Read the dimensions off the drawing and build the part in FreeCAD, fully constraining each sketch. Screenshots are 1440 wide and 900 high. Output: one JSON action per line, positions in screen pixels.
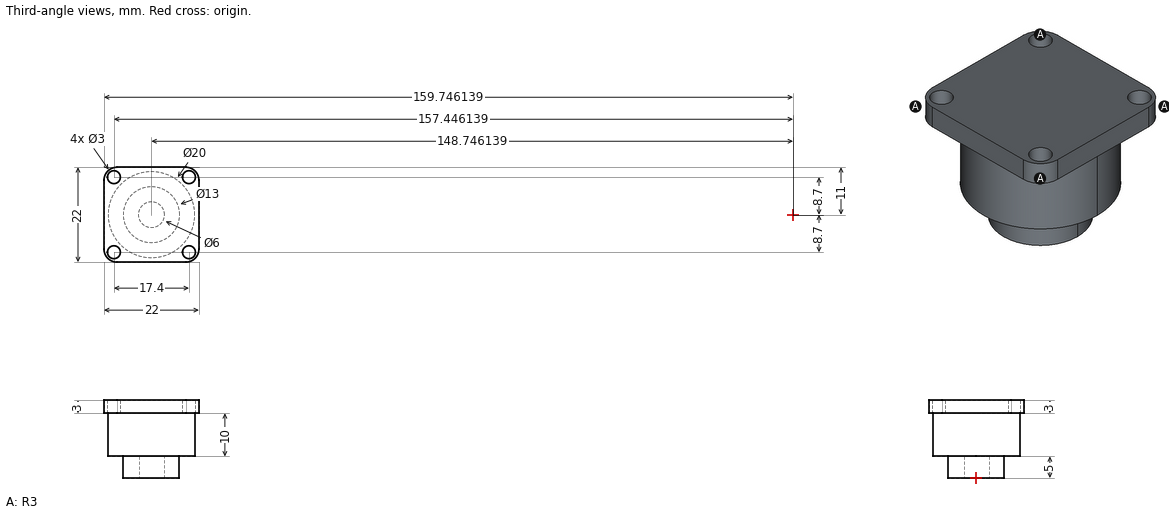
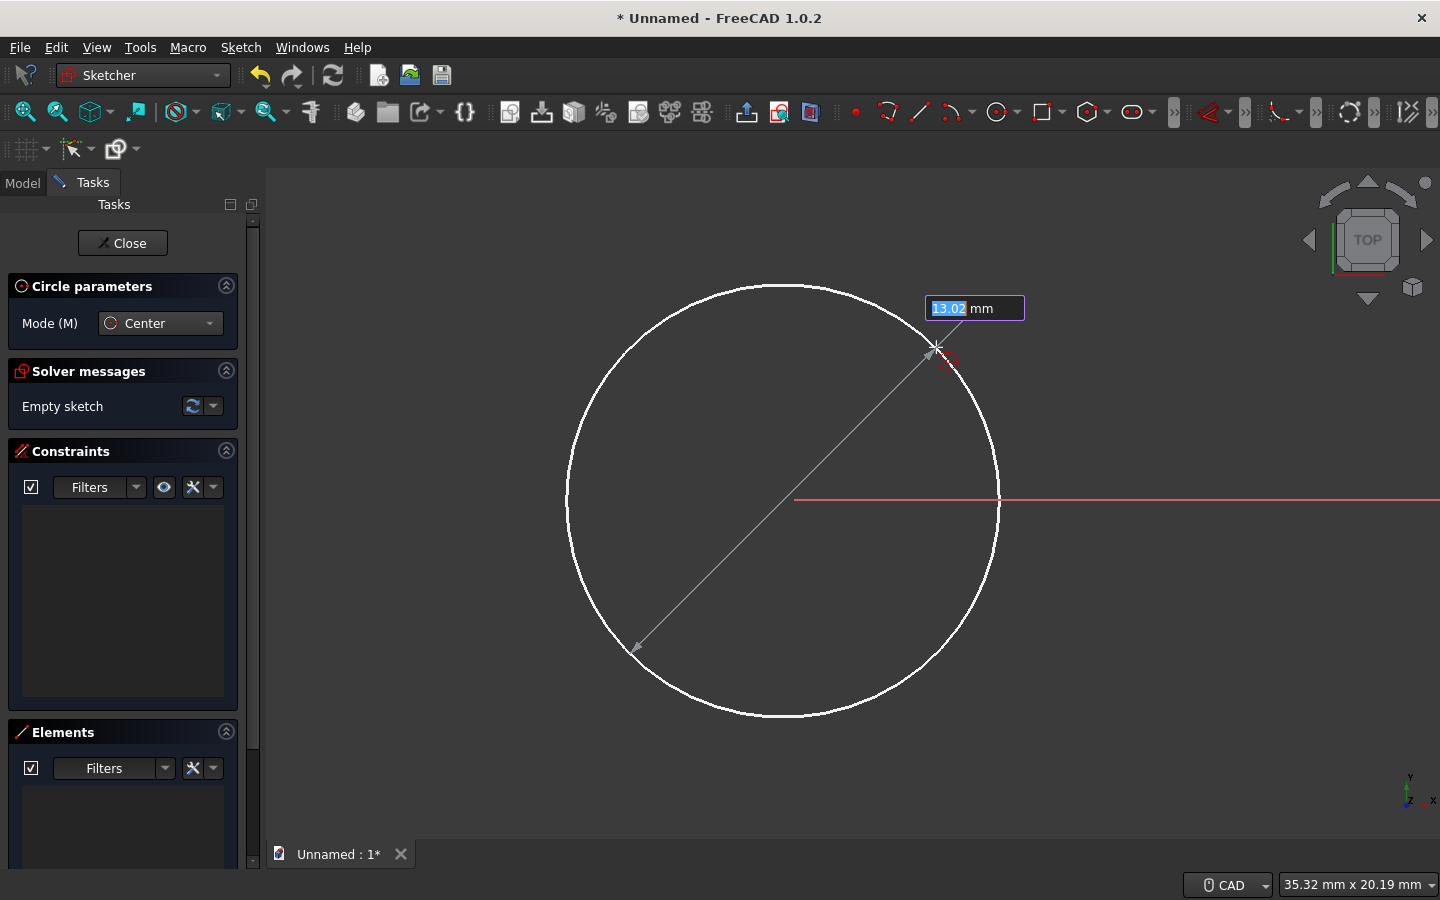
{"action": "type", "text": "13"}
{"action": "key", "text": "Return"}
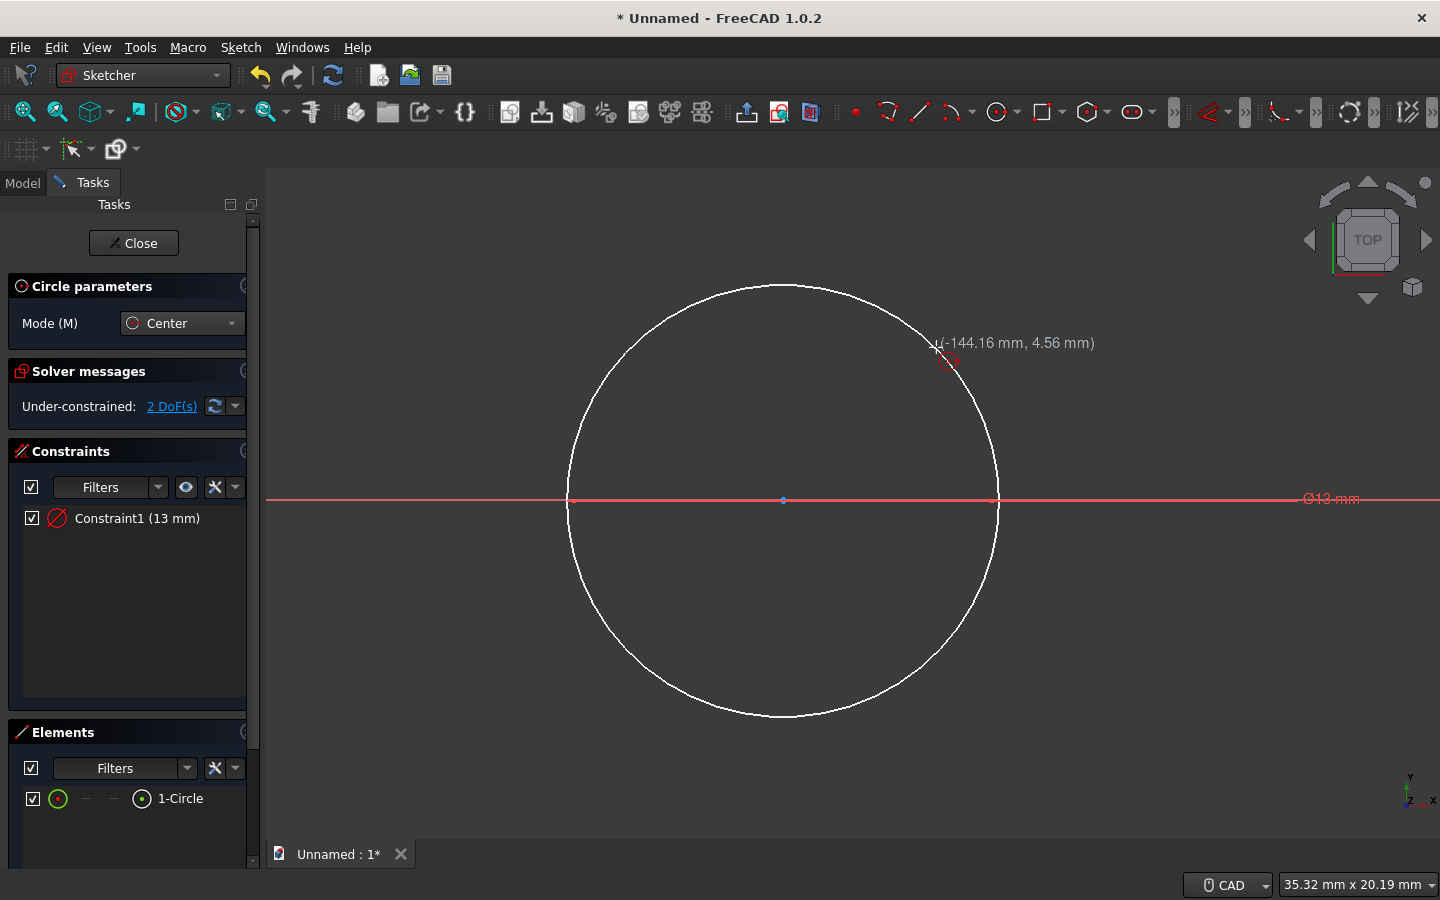
{"action": "left_click", "coordinate": [783, 501]}
{"action": "mouse_move", "coordinate": [854, 429]}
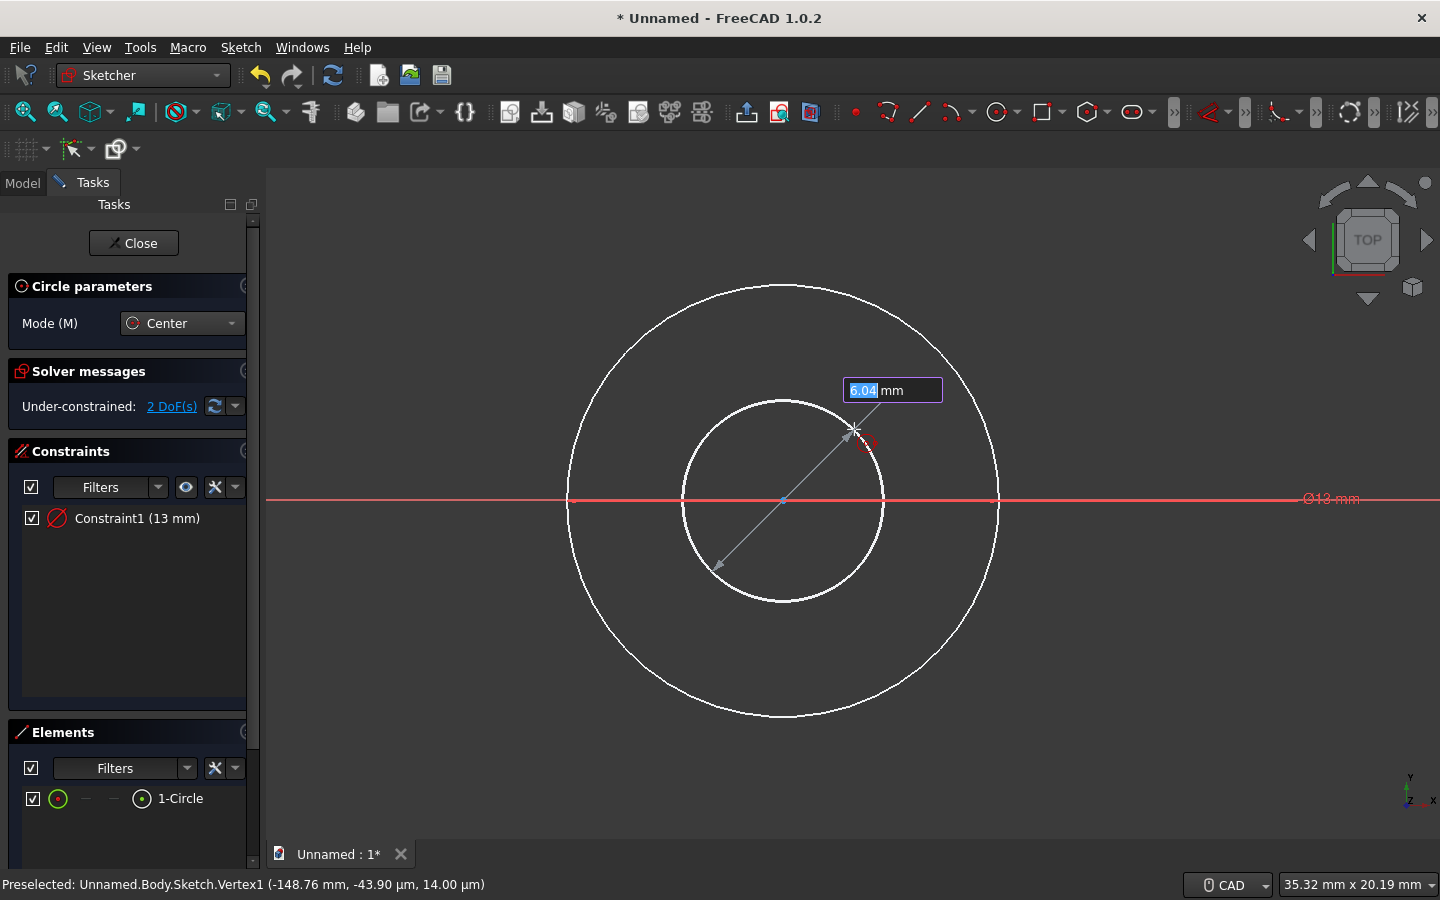
{"action": "type", "text": "6"}
{"action": "key", "text": "Return"}
{"action": "key", "text": "Escape"}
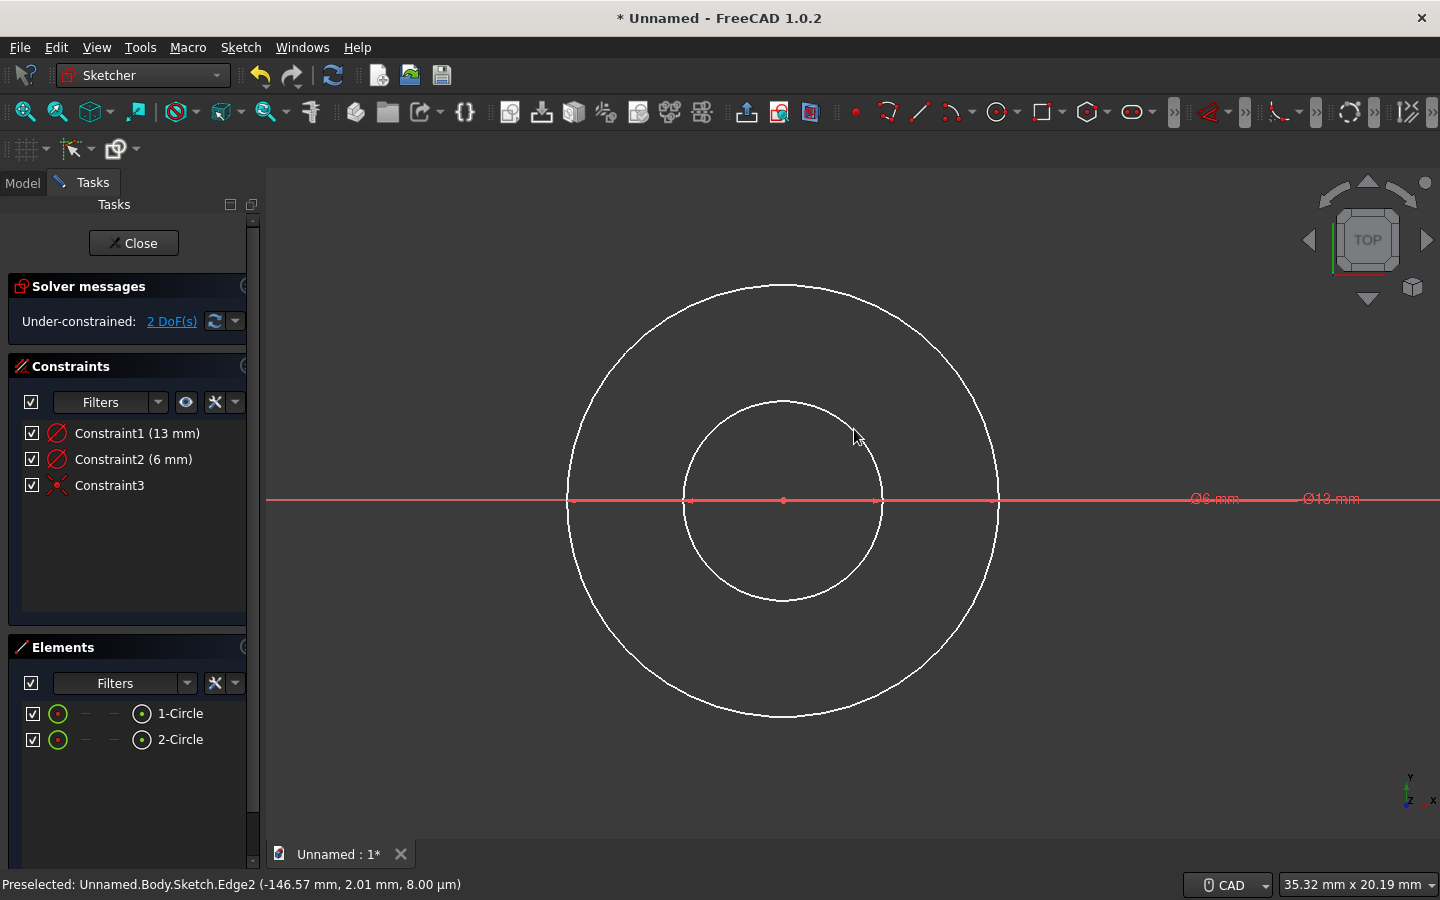
{"action": "left_click", "coordinate": [783, 501]}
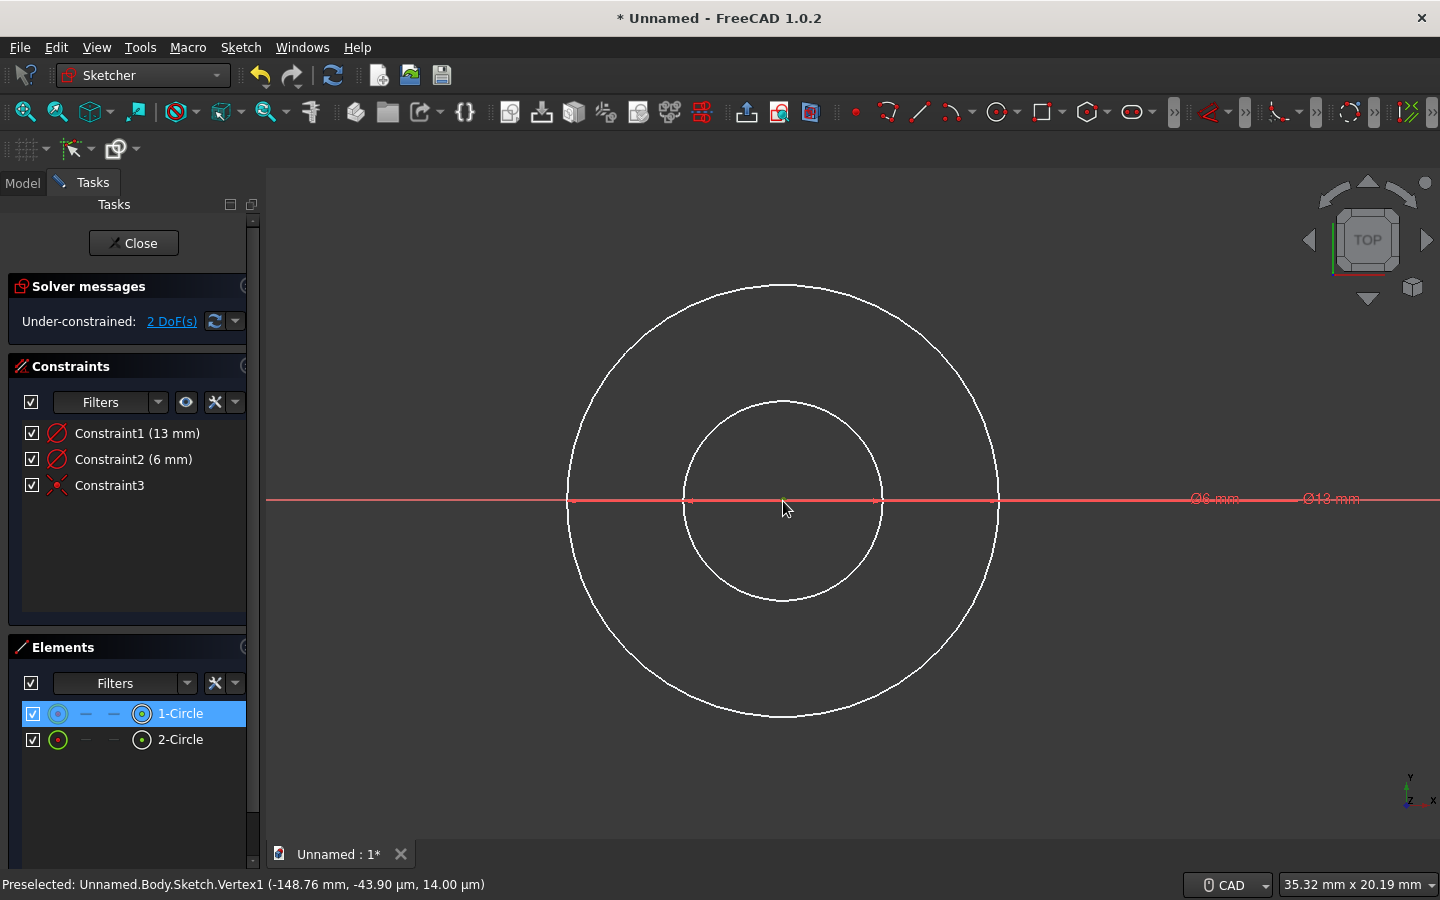
{"action": "left_click", "coordinate": [364, 500]}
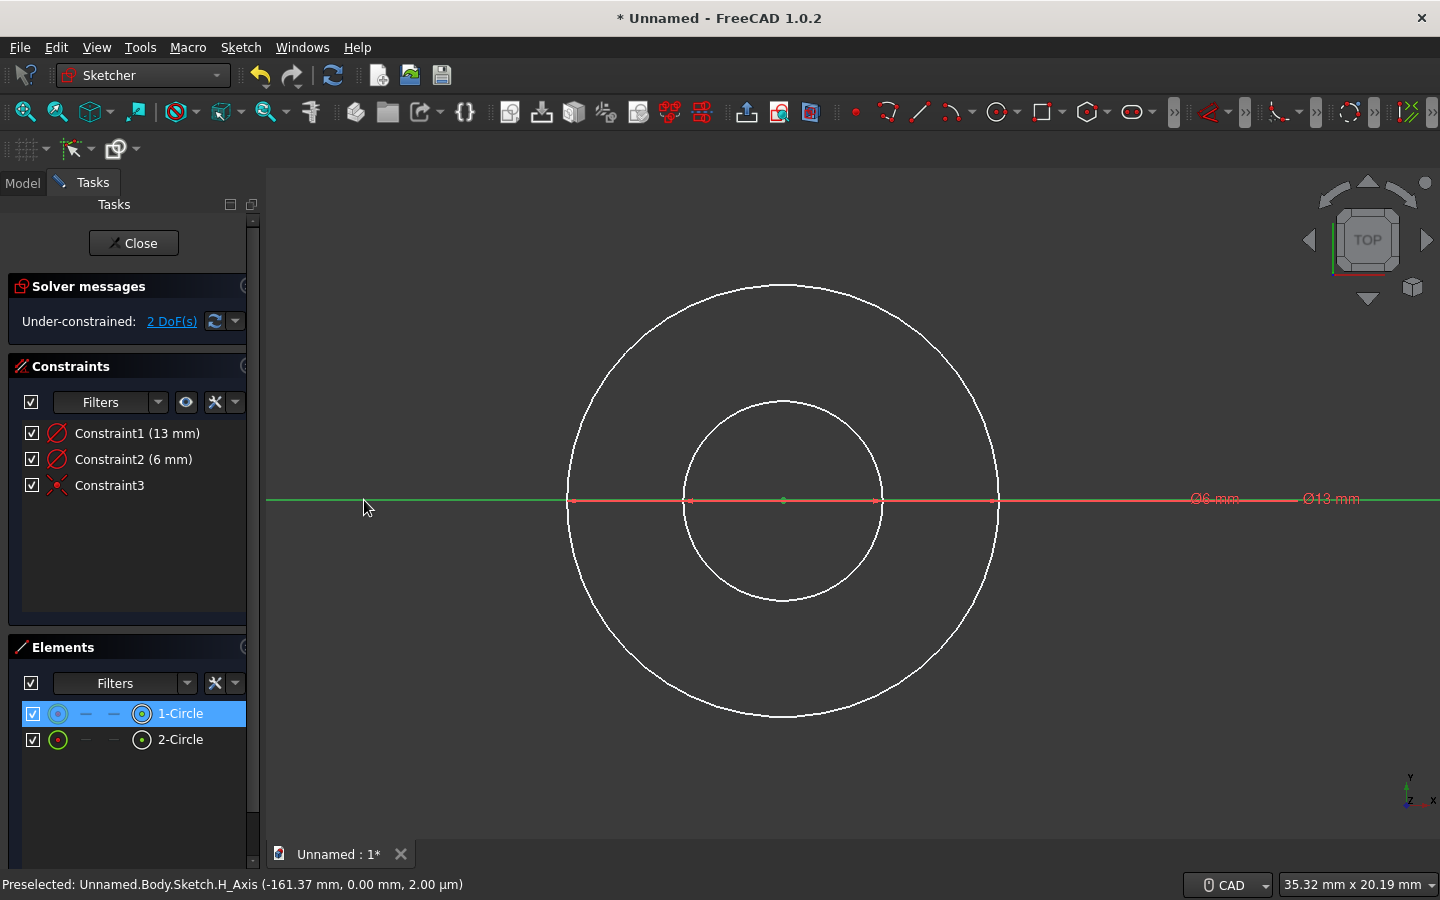
{"action": "key", "text": "c"}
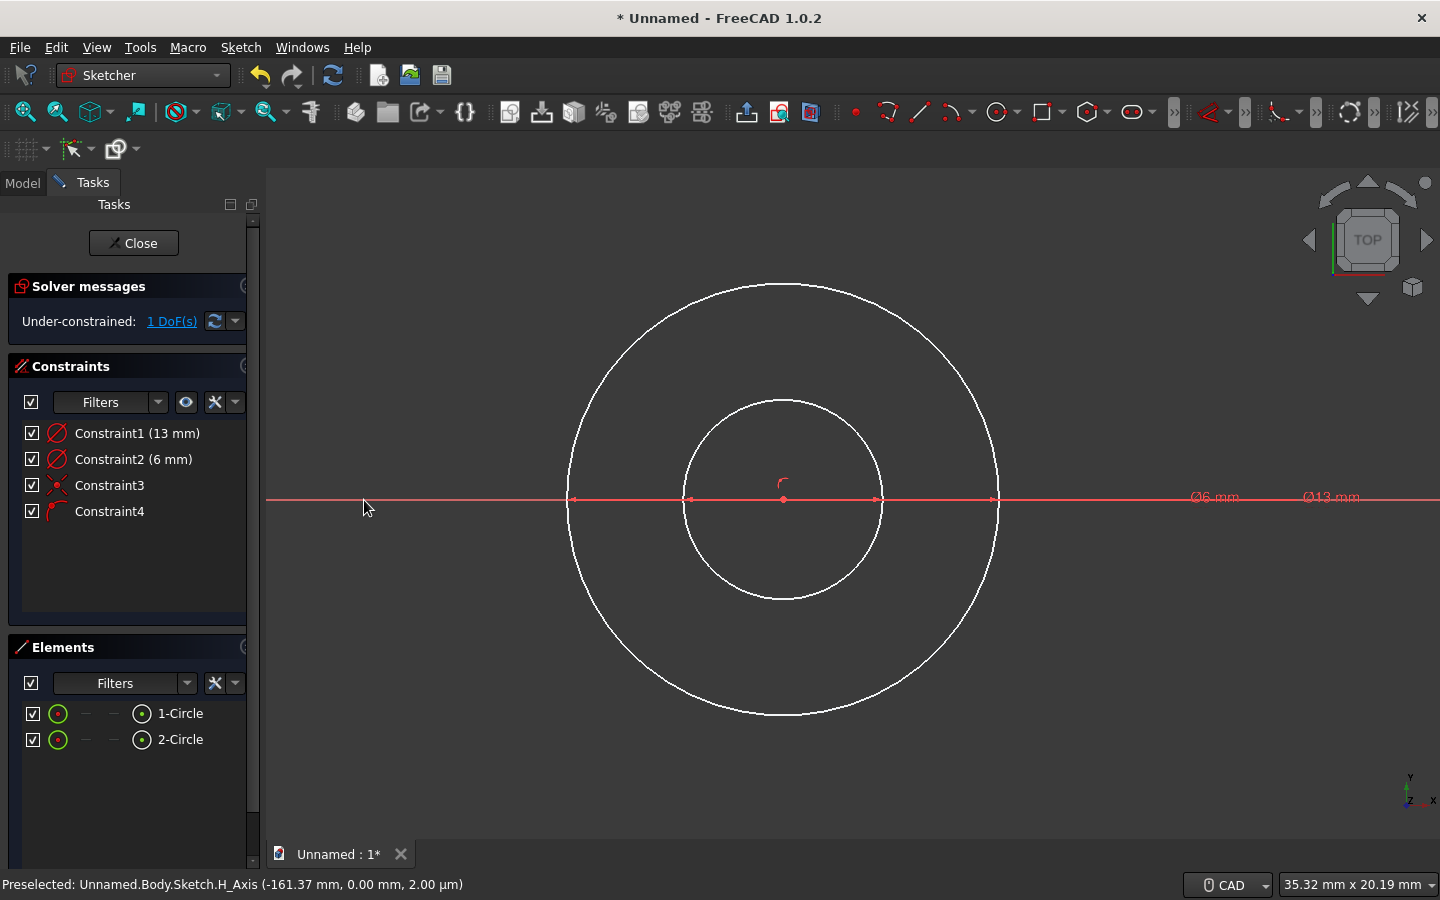
{"action": "left_click", "coordinate": [1208, 112]}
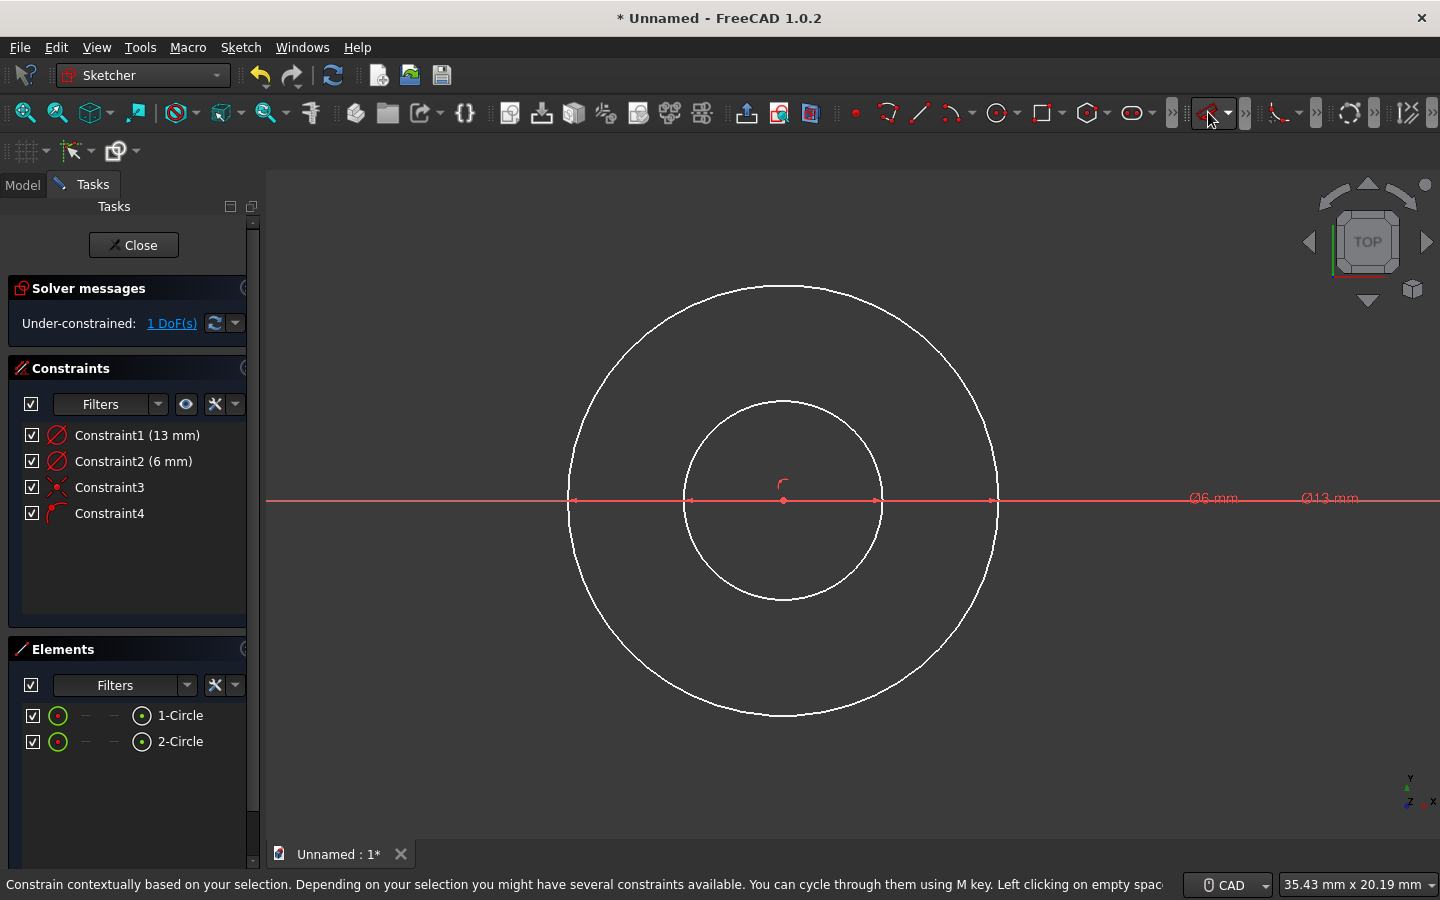
{"action": "left_click", "coordinate": [783, 501]}
{"action": "left_click", "coordinate": [1029, 535]}